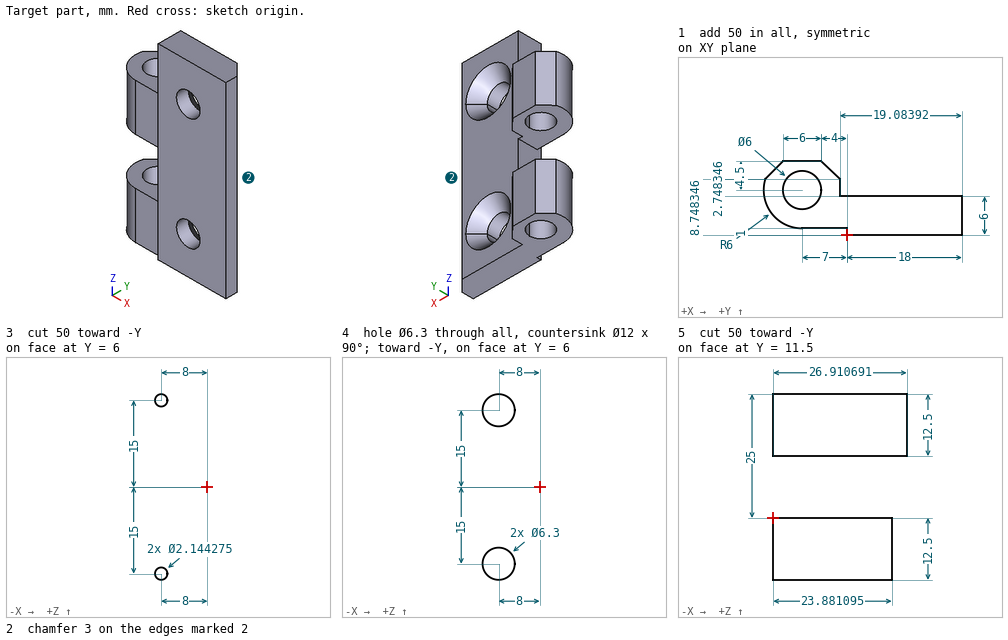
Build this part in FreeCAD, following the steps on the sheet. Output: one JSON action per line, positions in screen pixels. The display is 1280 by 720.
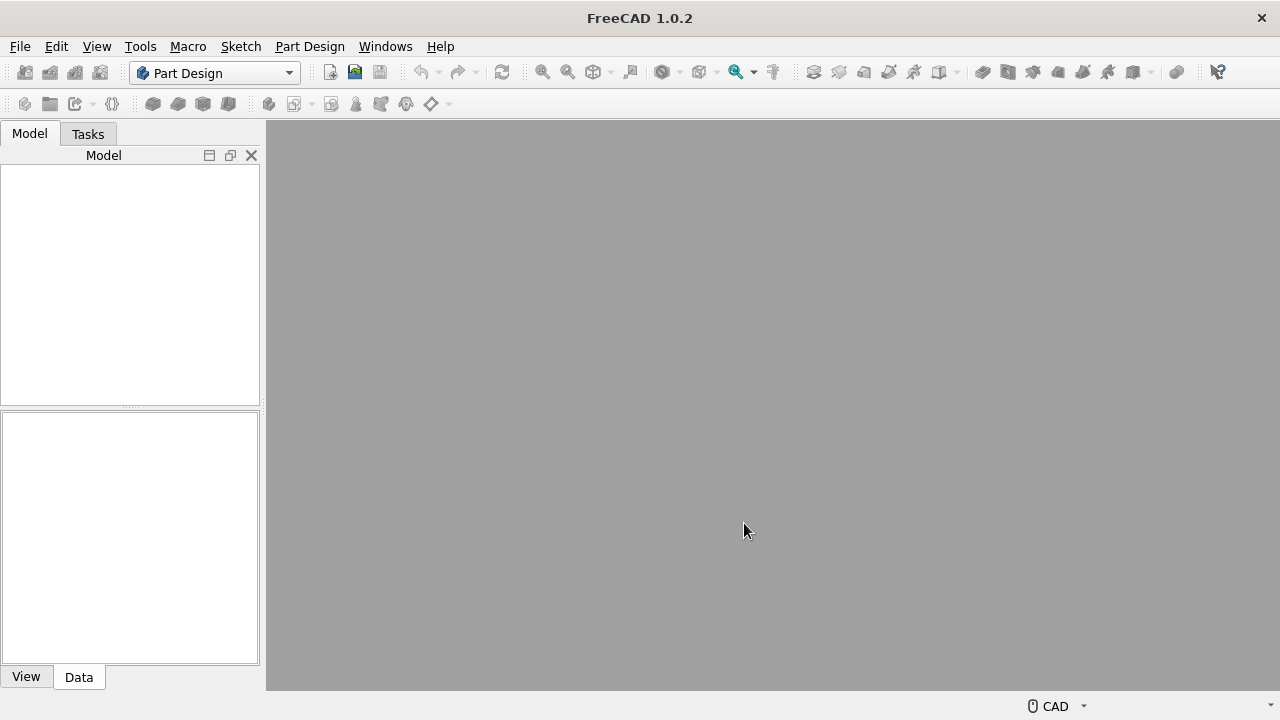
{"action": "left_click", "coordinate": [330, 72]}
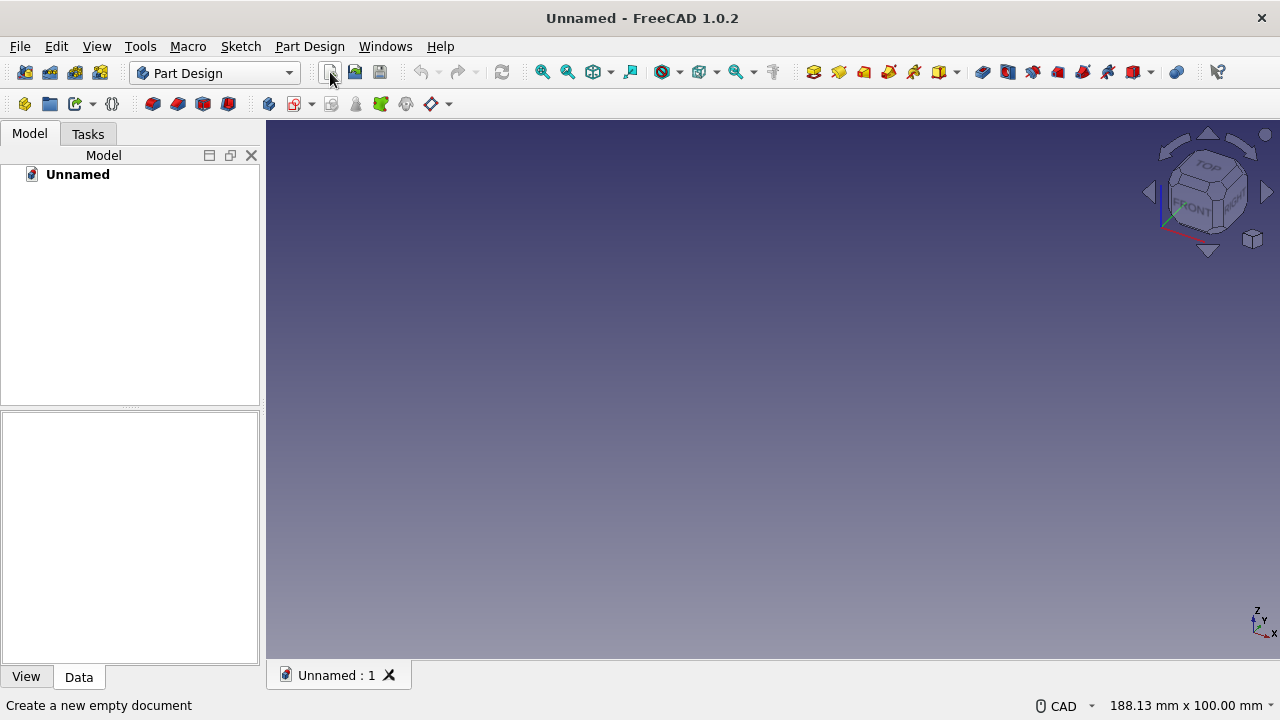
{"action": "left_click", "coordinate": [294, 104]}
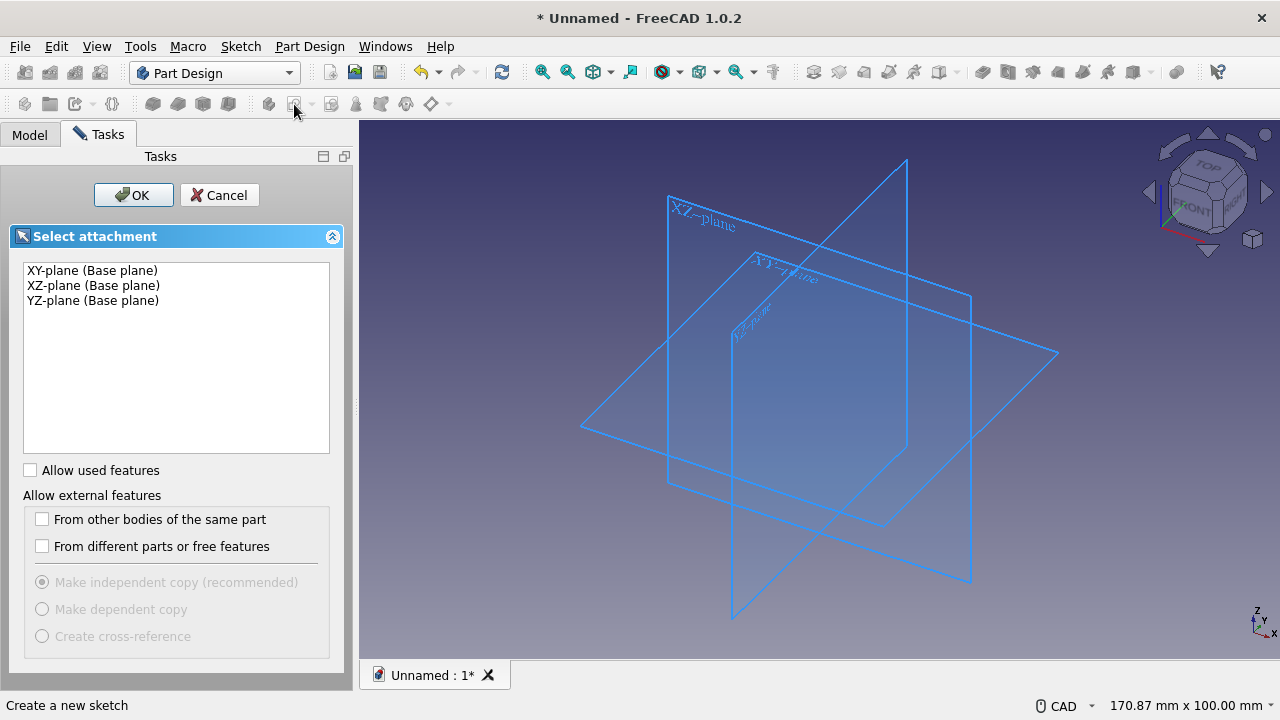
{"action": "left_click", "coordinate": [84, 270]}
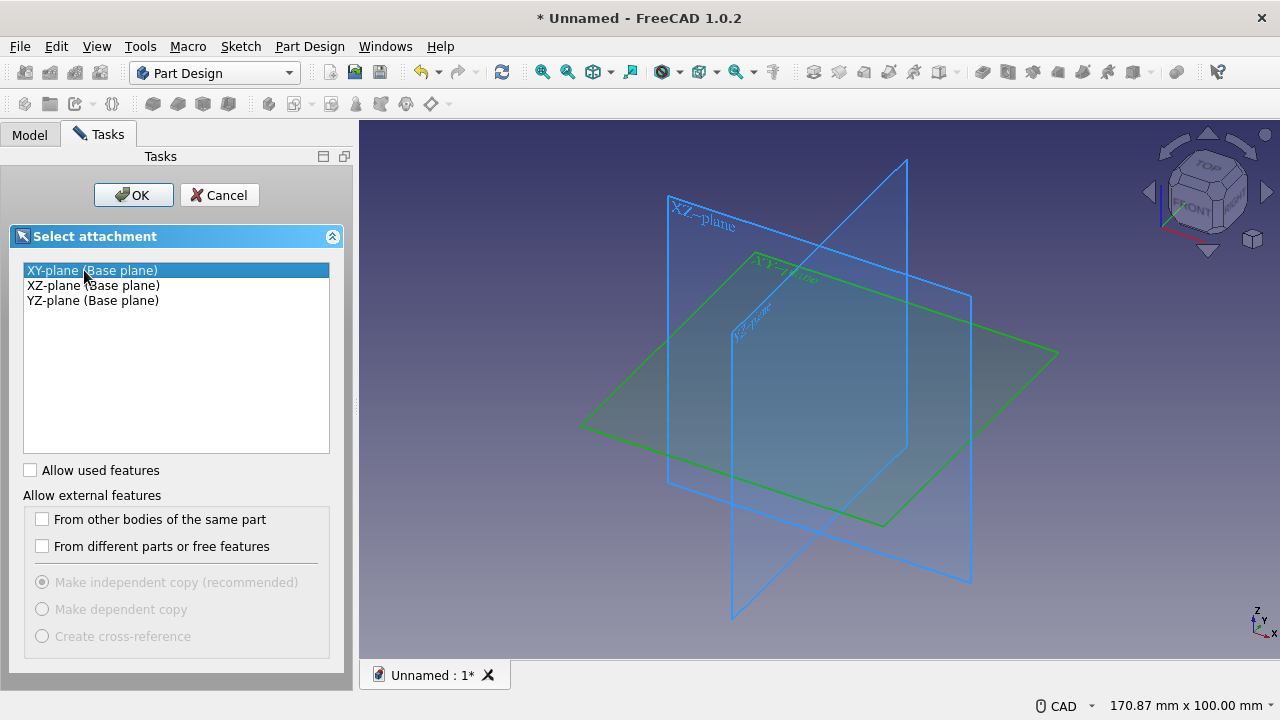
{"action": "left_click", "coordinate": [134, 195]}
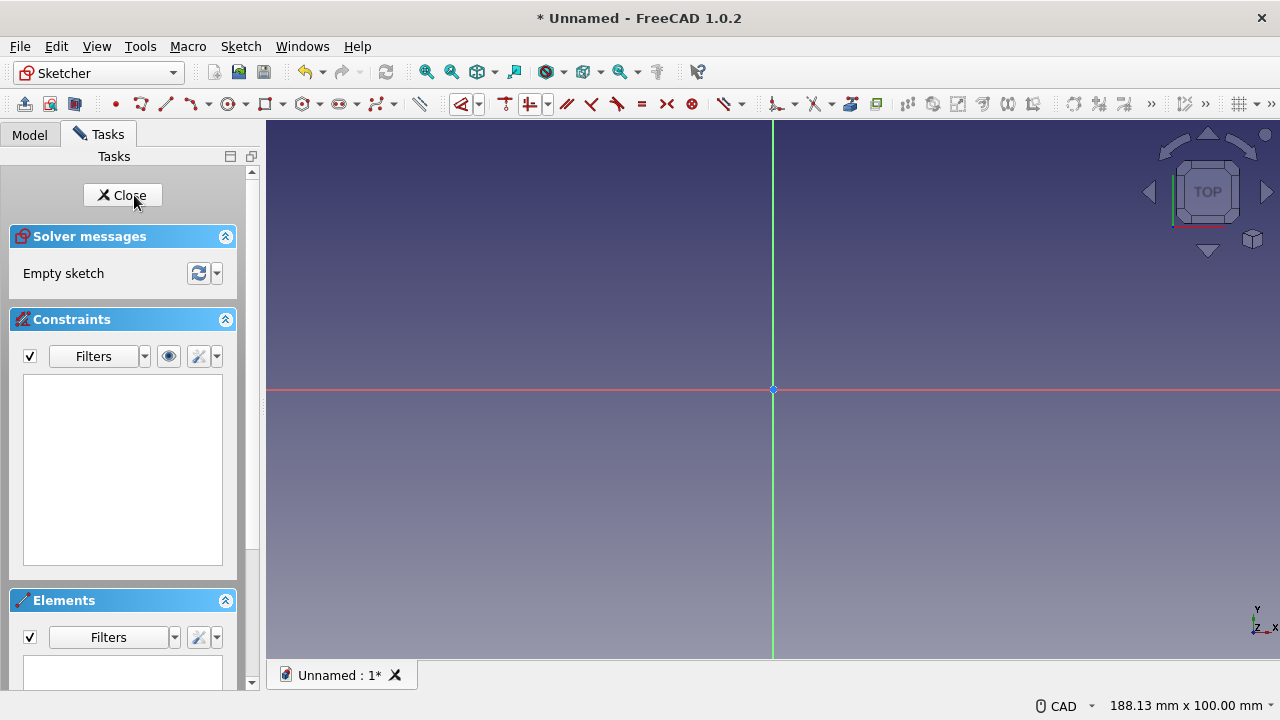
{"action": "scroll", "coordinate": [823, 345], "scroll_direction": "up", "scroll_amount": 6}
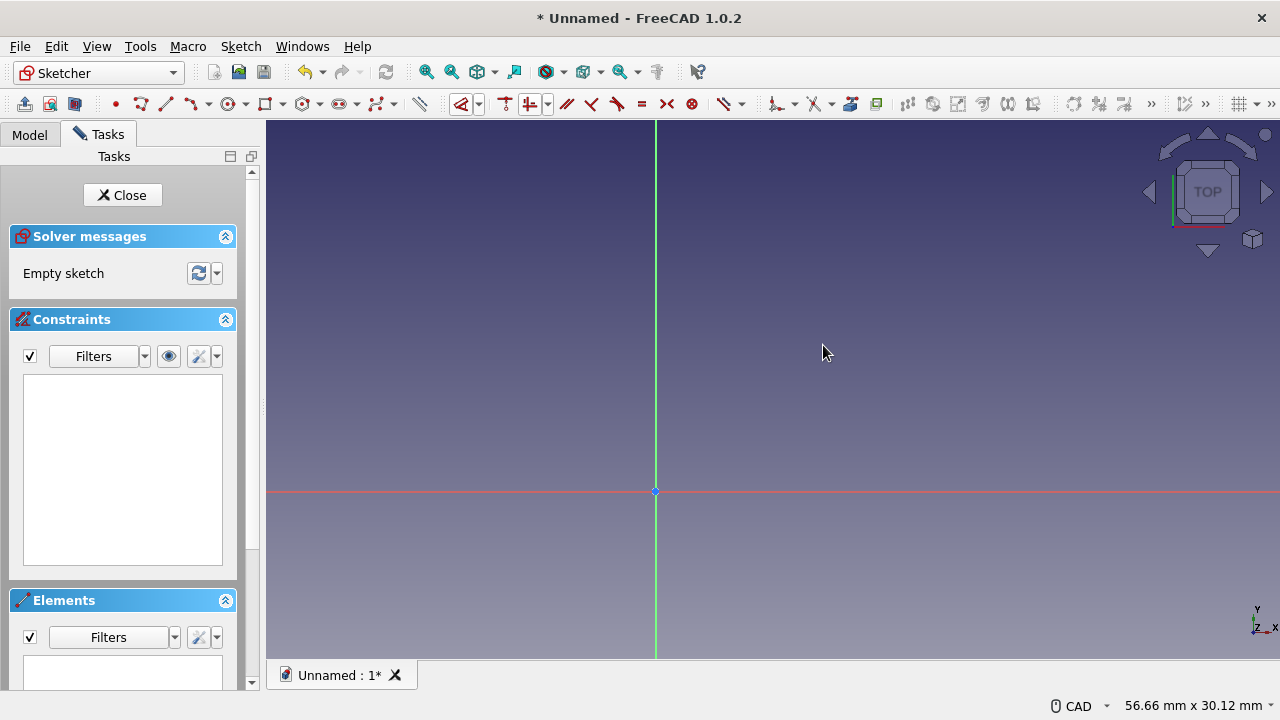
{"action": "left_click", "coordinate": [141, 104]}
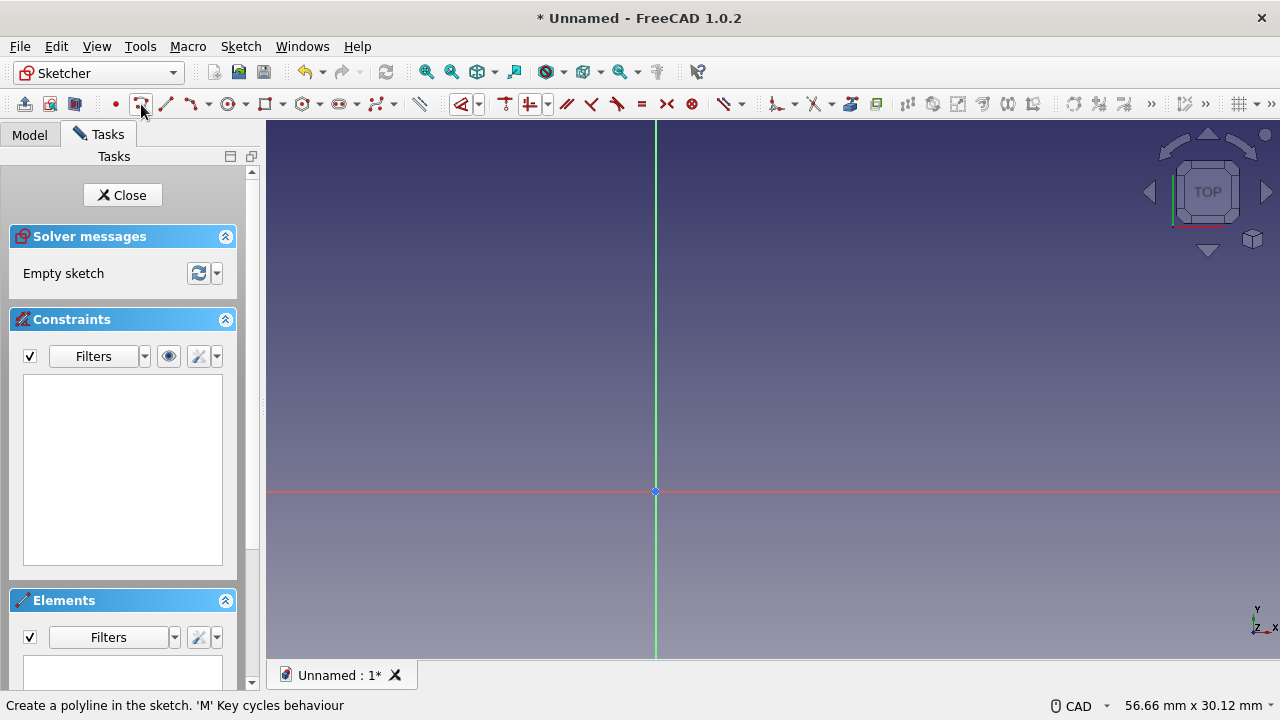
{"action": "left_click", "coordinate": [530, 474]}
{"action": "left_click", "coordinate": [656, 474]}
{"action": "left_click", "coordinate": [656, 492]}
{"action": "left_click", "coordinate": [978, 483]}
{"action": "left_click", "coordinate": [978, 384]}
{"action": "left_click", "coordinate": [636, 384]}
{"action": "left_click", "coordinate": [636, 335]}
{"action": "left_click", "coordinate": [584, 286]}
{"action": "left_click", "coordinate": [477, 286]}
{"action": "left_click", "coordinate": [428, 335]}
{"action": "right_click", "coordinate": [428, 335]}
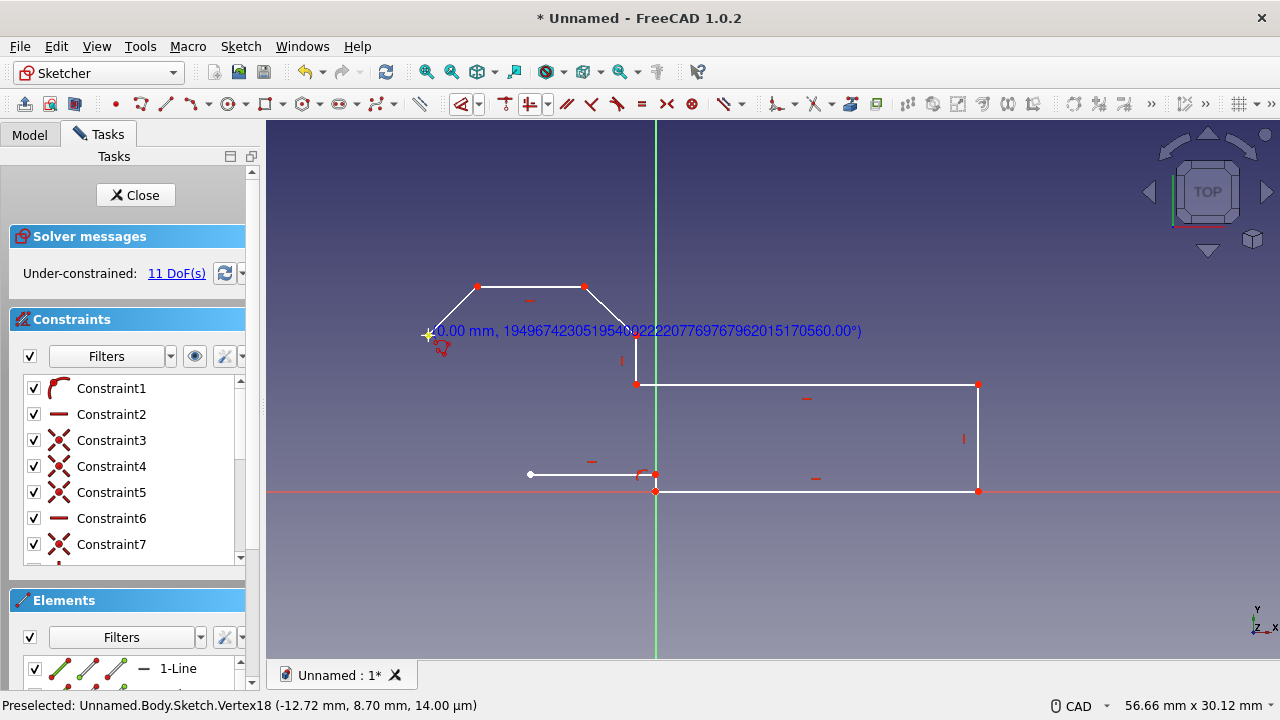
{"action": "left_click", "coordinate": [190, 104]}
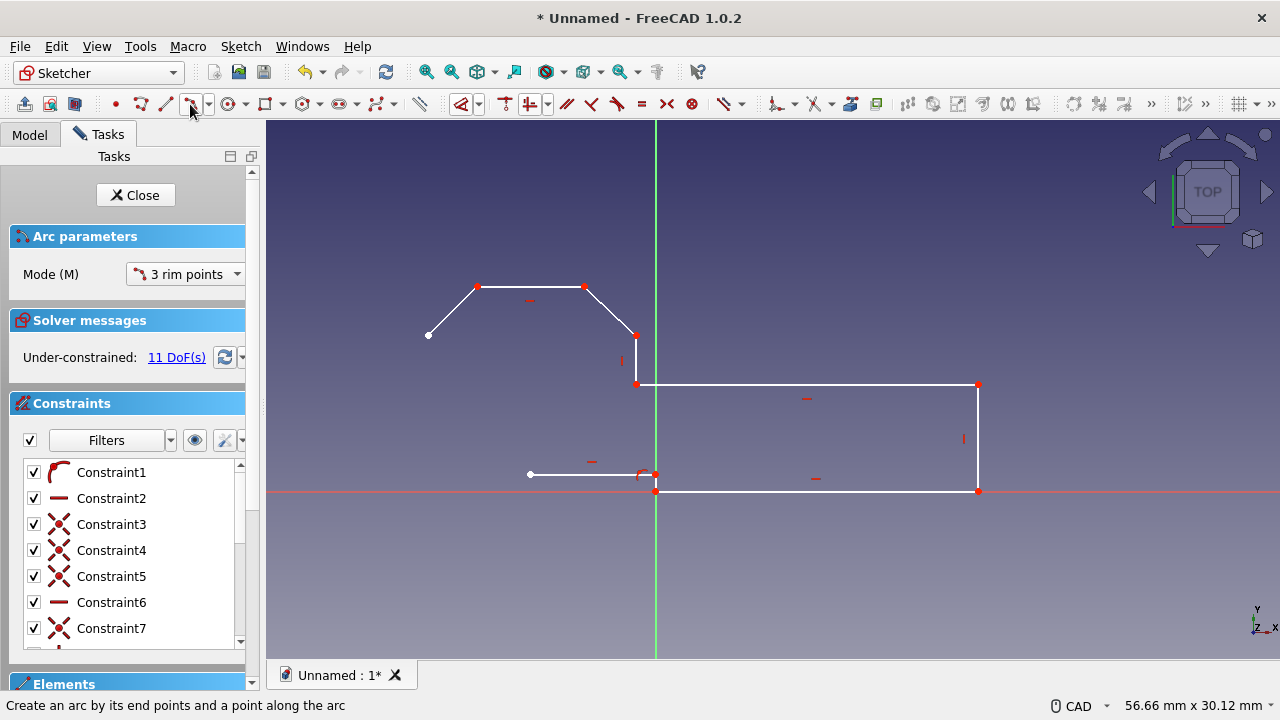
{"action": "left_click", "coordinate": [428, 336]}
{"action": "left_click", "coordinate": [530, 475]}
{"action": "left_click", "coordinate": [444, 430]}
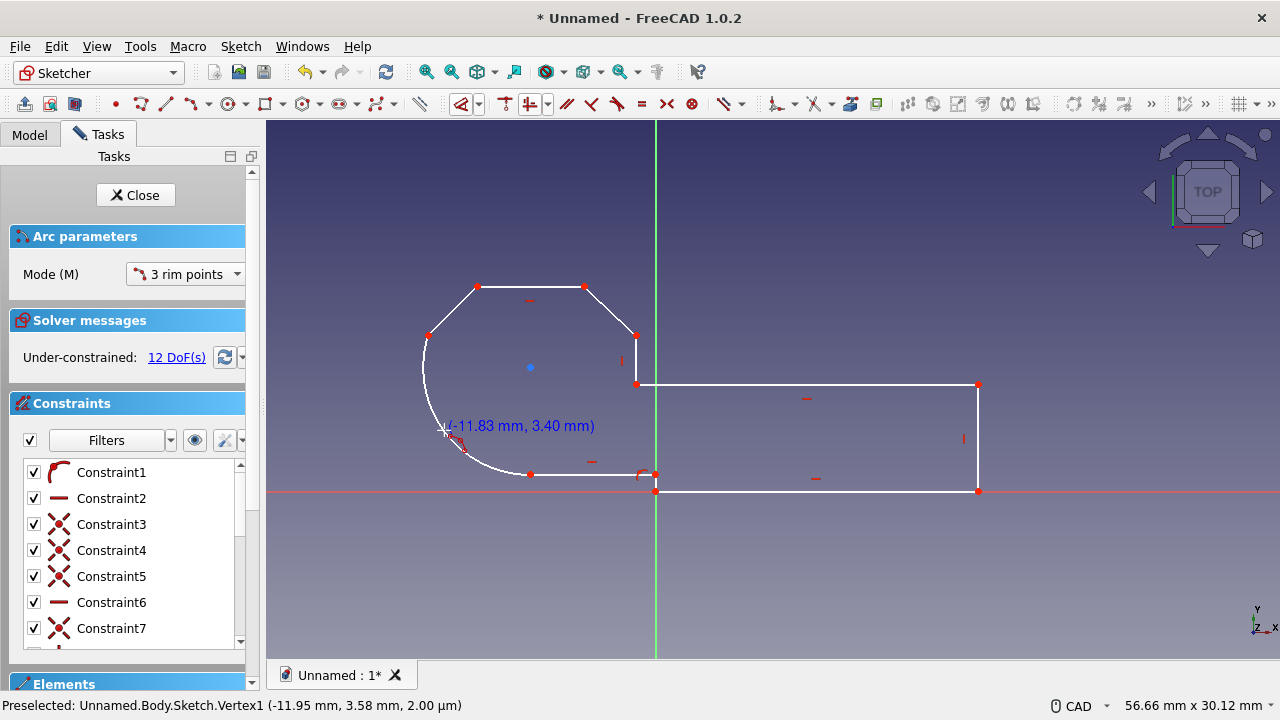
{"action": "key", "text": "g c"}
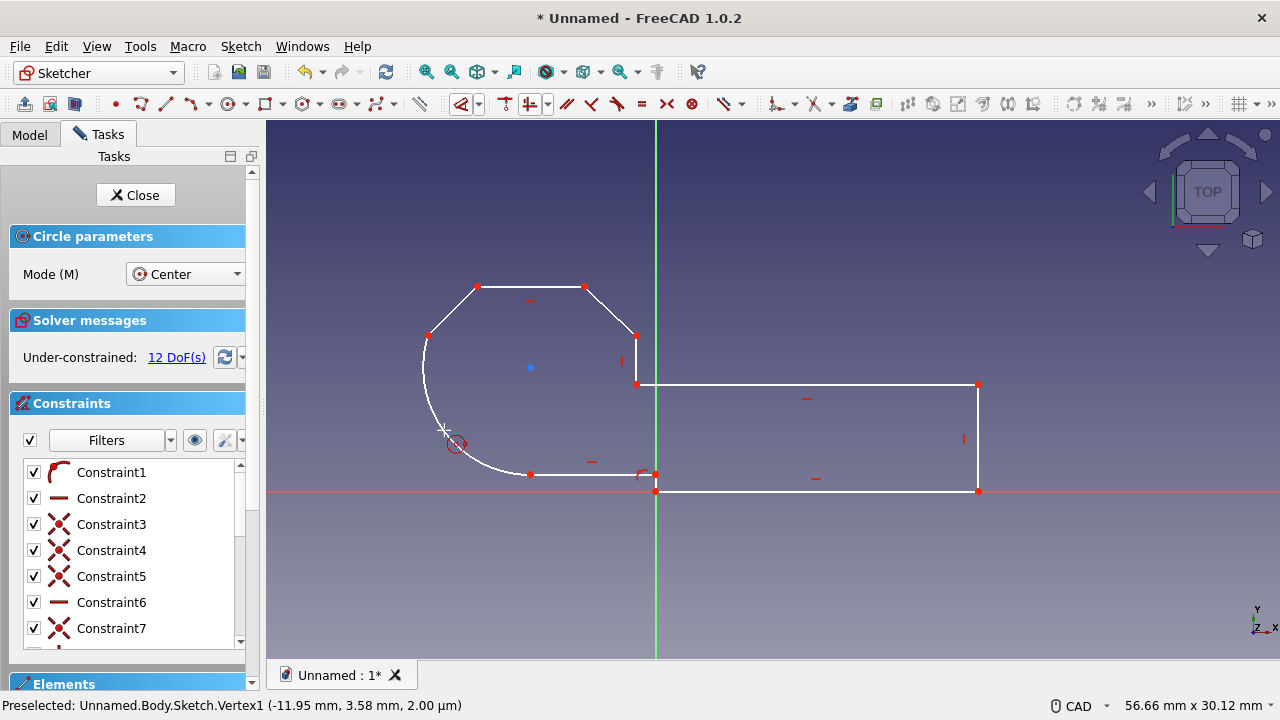
{"action": "left_click", "coordinate": [530, 367]}
{"action": "mouse_move", "coordinate": [568, 329]}